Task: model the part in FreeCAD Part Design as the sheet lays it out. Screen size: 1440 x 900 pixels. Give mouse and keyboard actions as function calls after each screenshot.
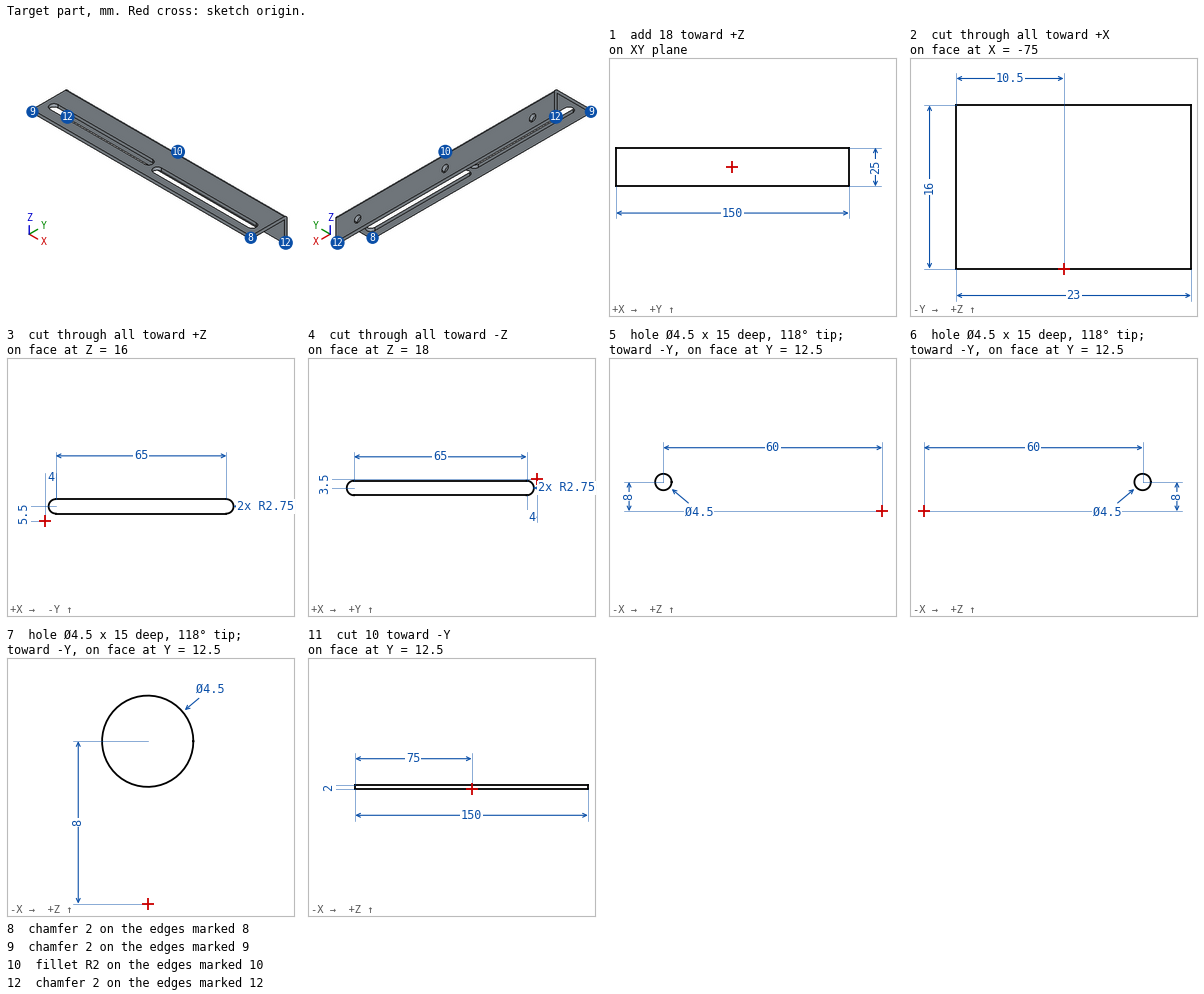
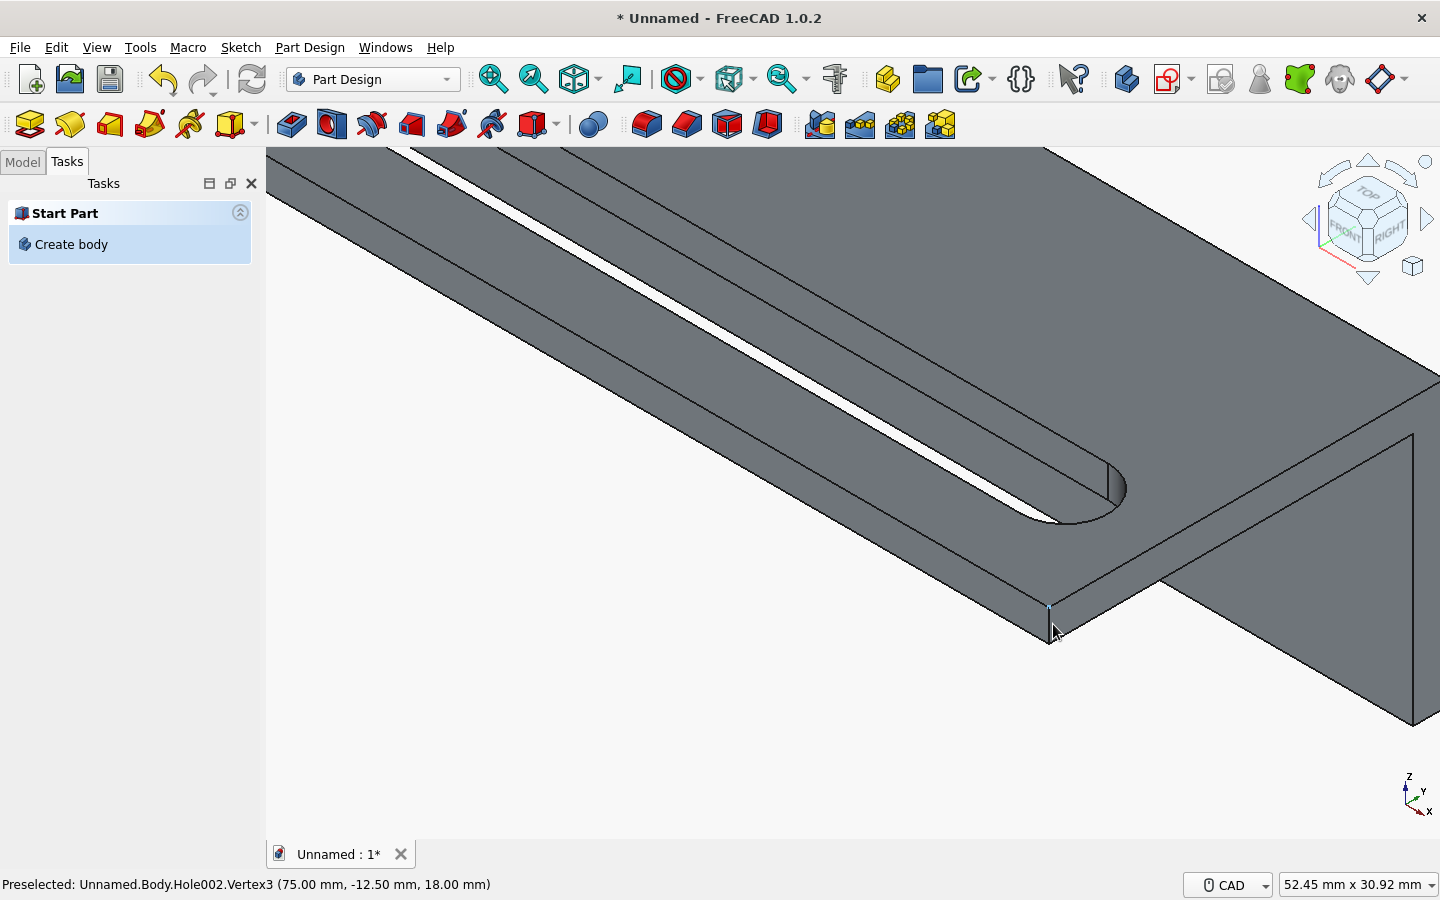
click(1049, 625)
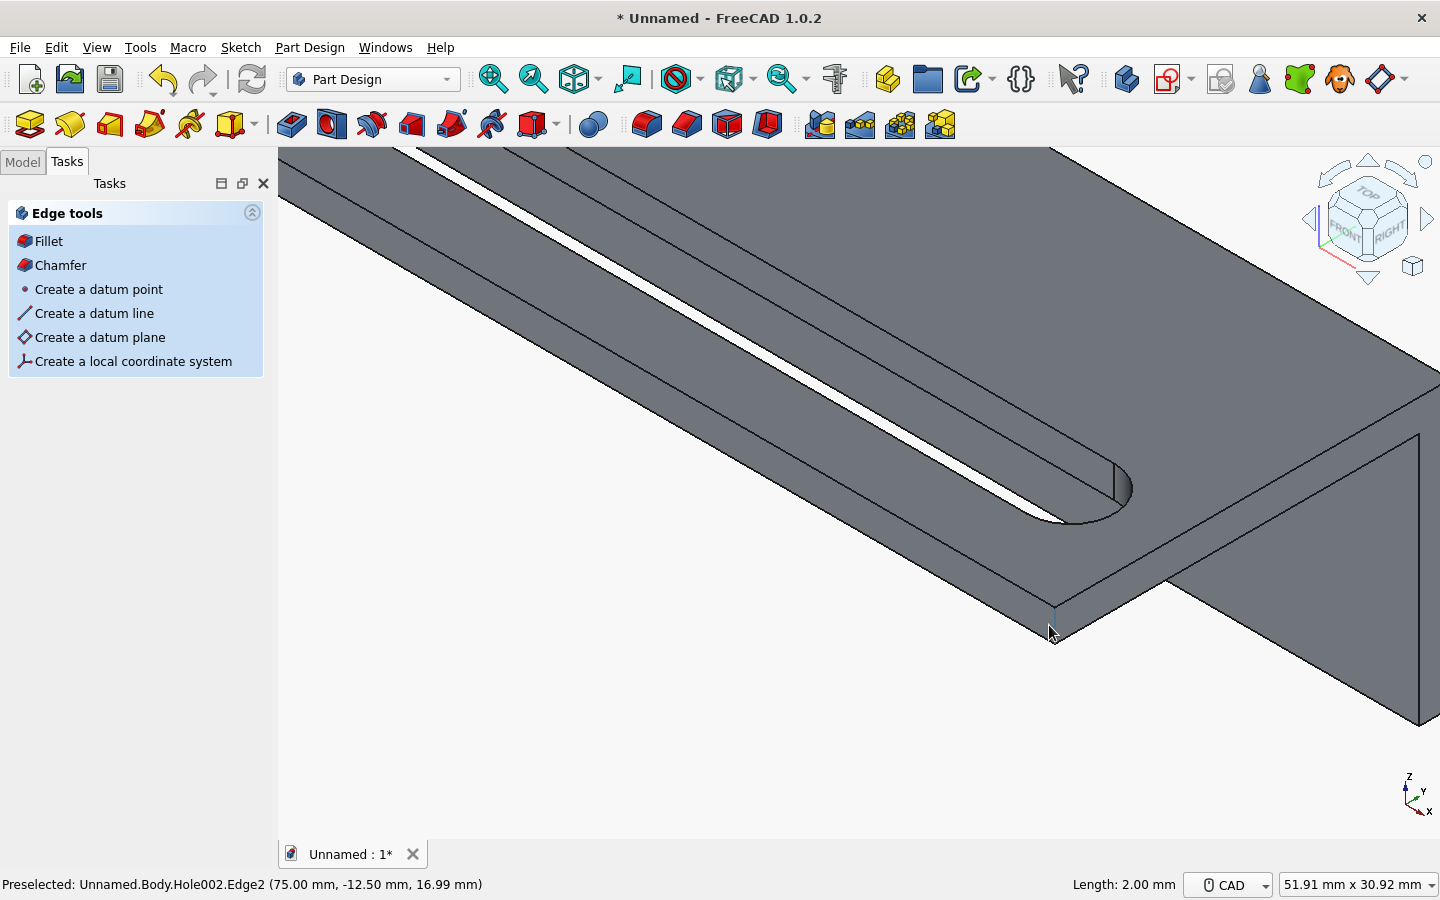
click(688, 124)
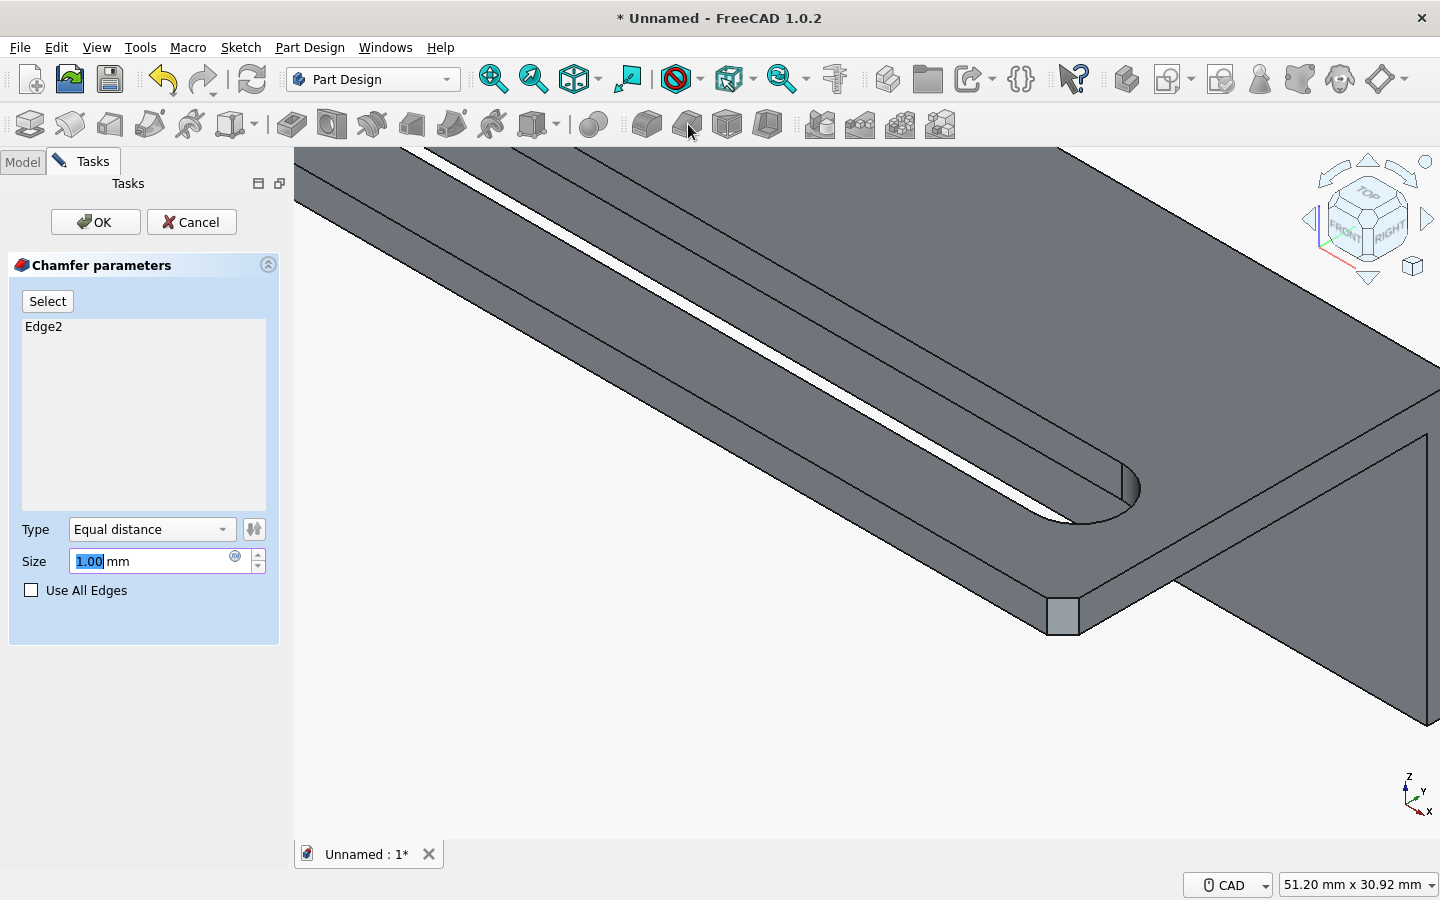
text(2)
key(Tab)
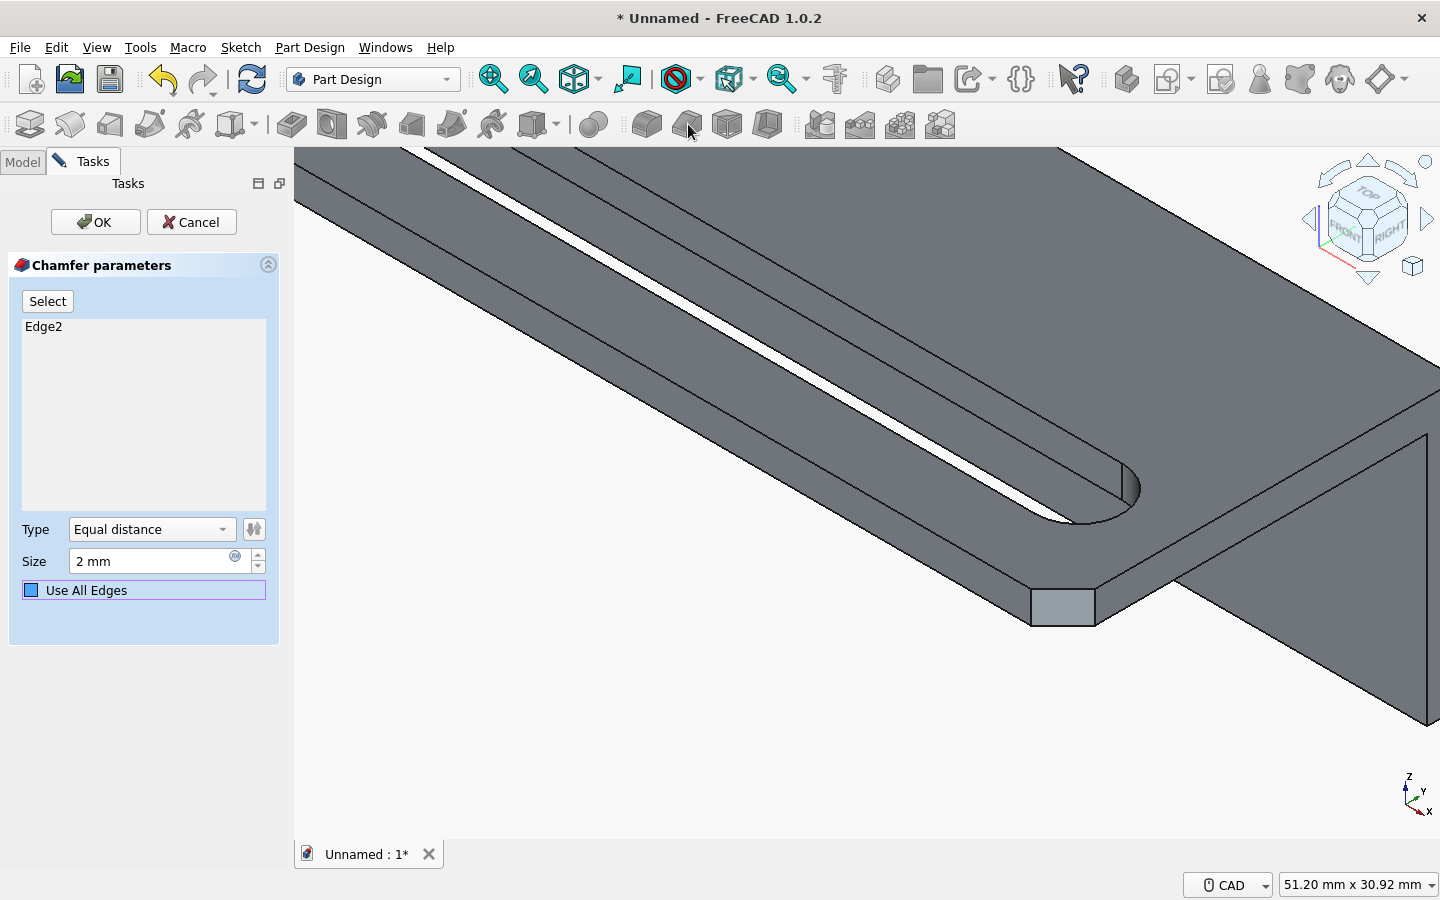
click(96, 222)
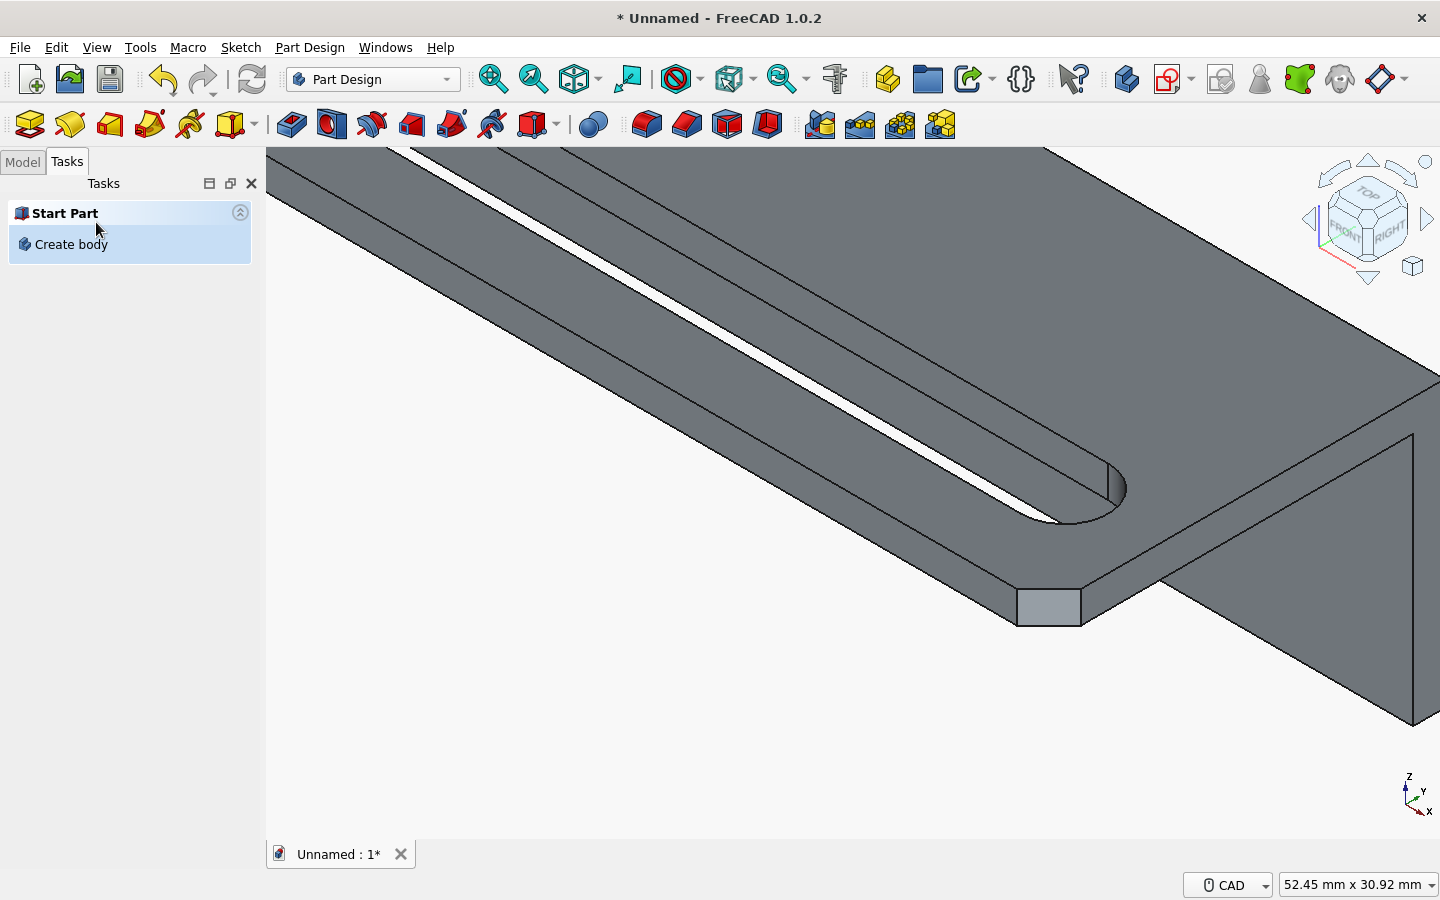
click(494, 80)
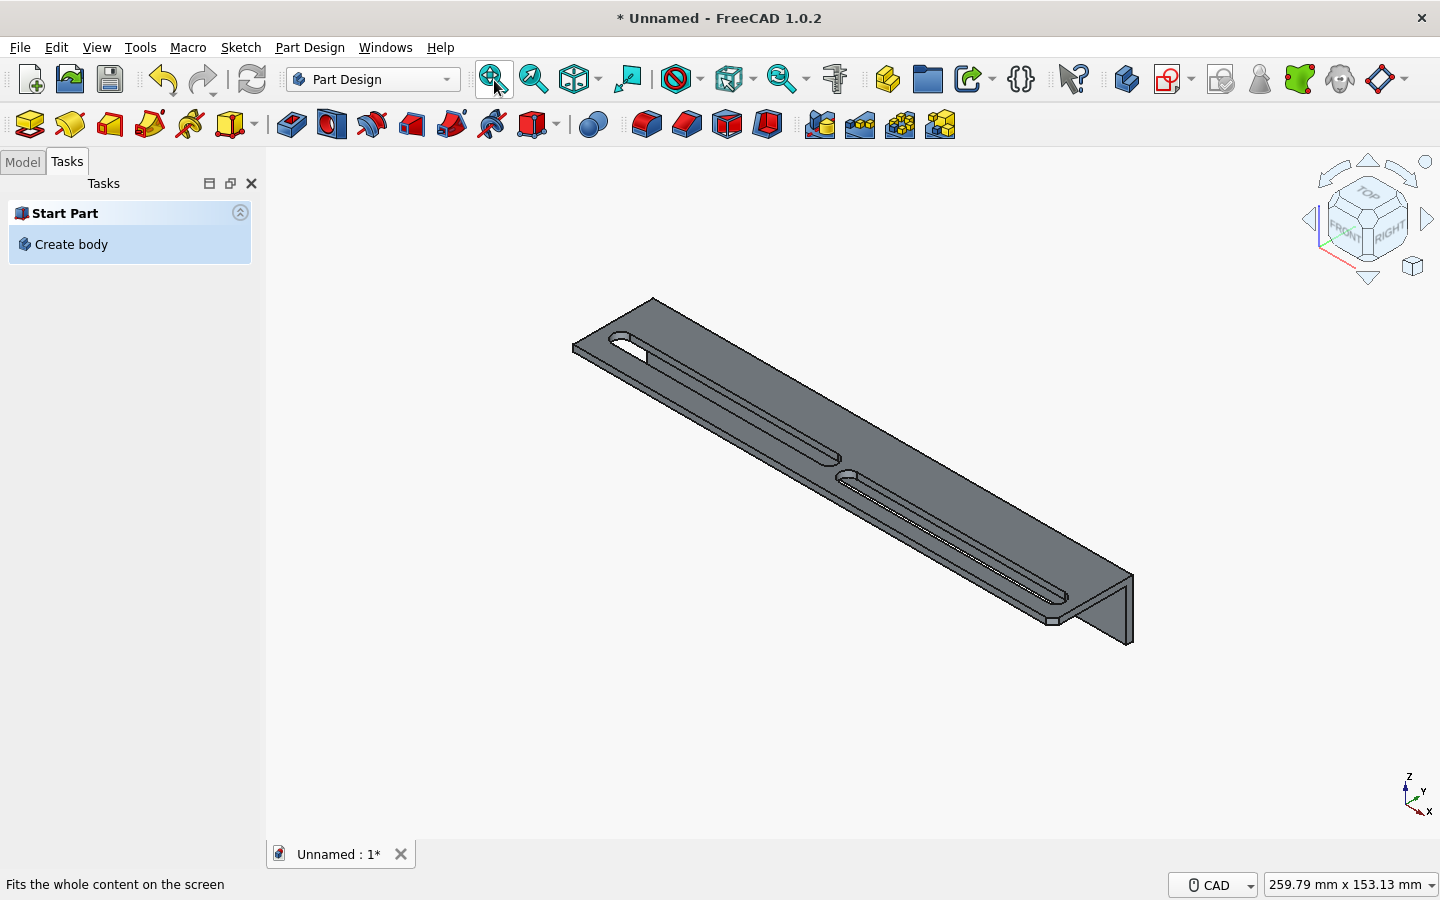
scroll(573, 347, up, 8)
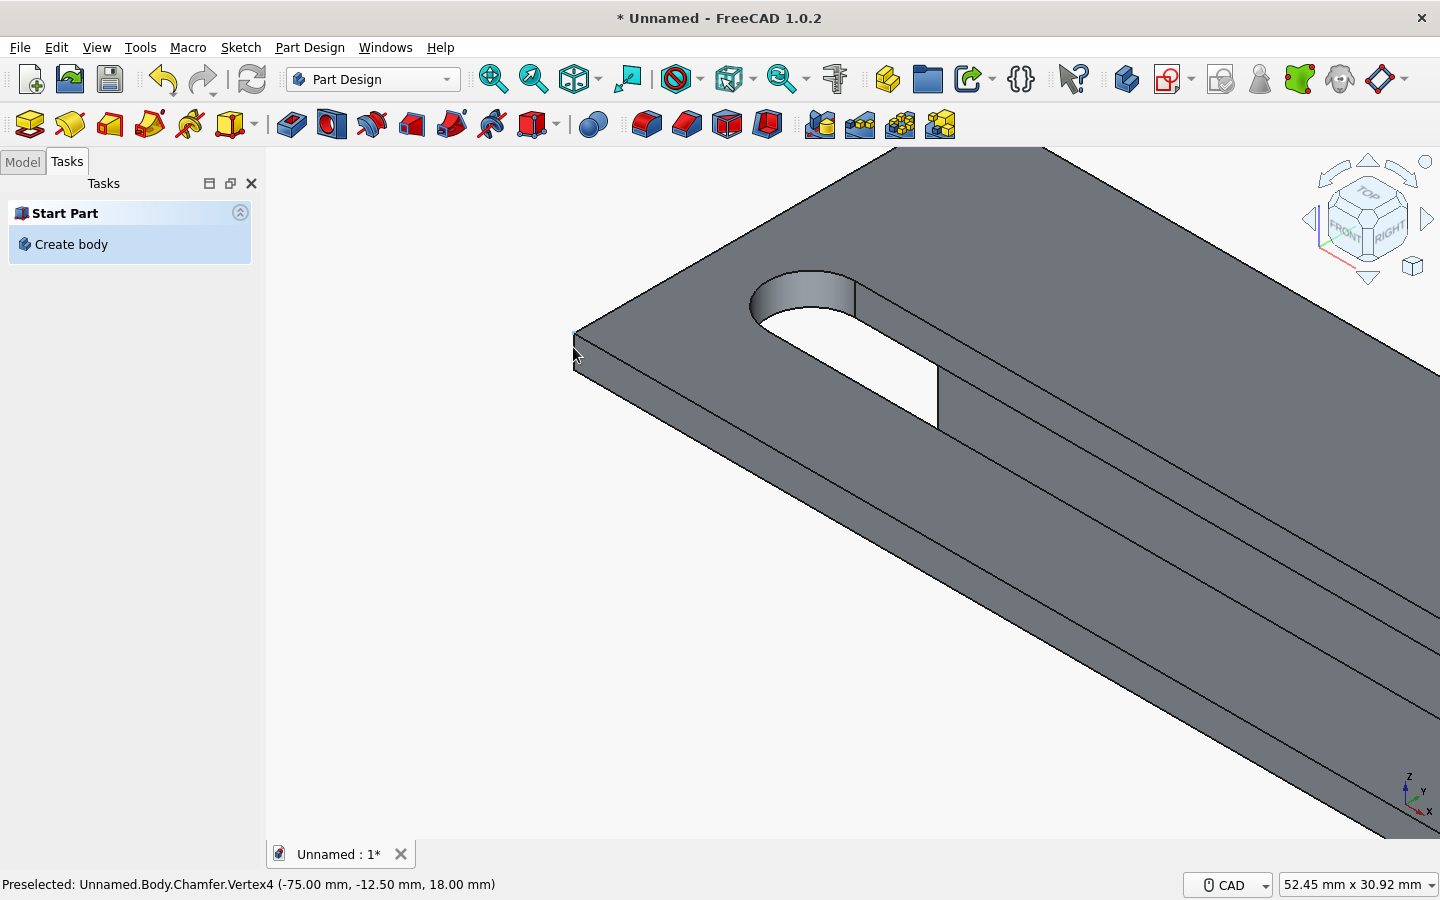
click(494, 80)